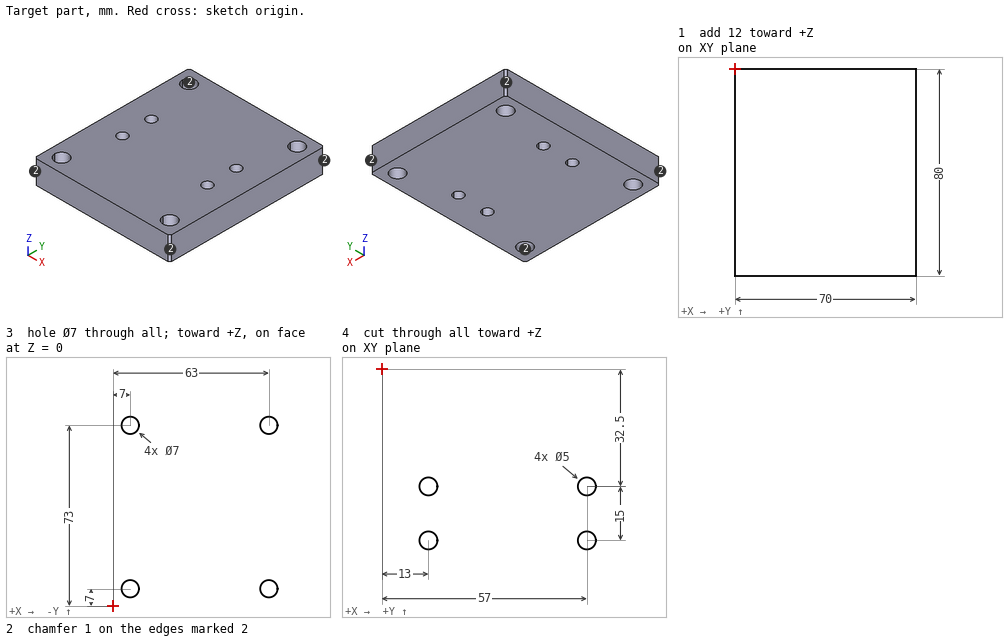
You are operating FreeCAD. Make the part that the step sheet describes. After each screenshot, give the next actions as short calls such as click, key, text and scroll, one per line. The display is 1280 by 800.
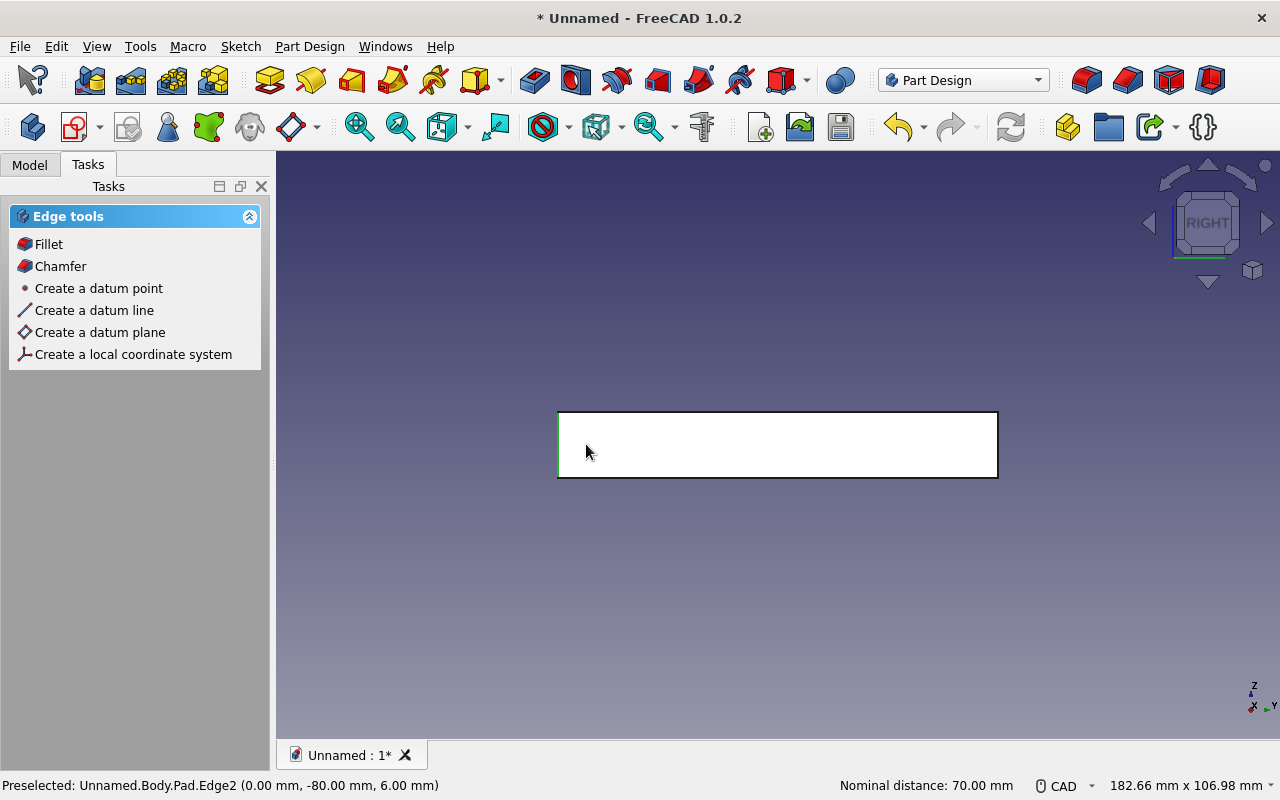
click(360, 128)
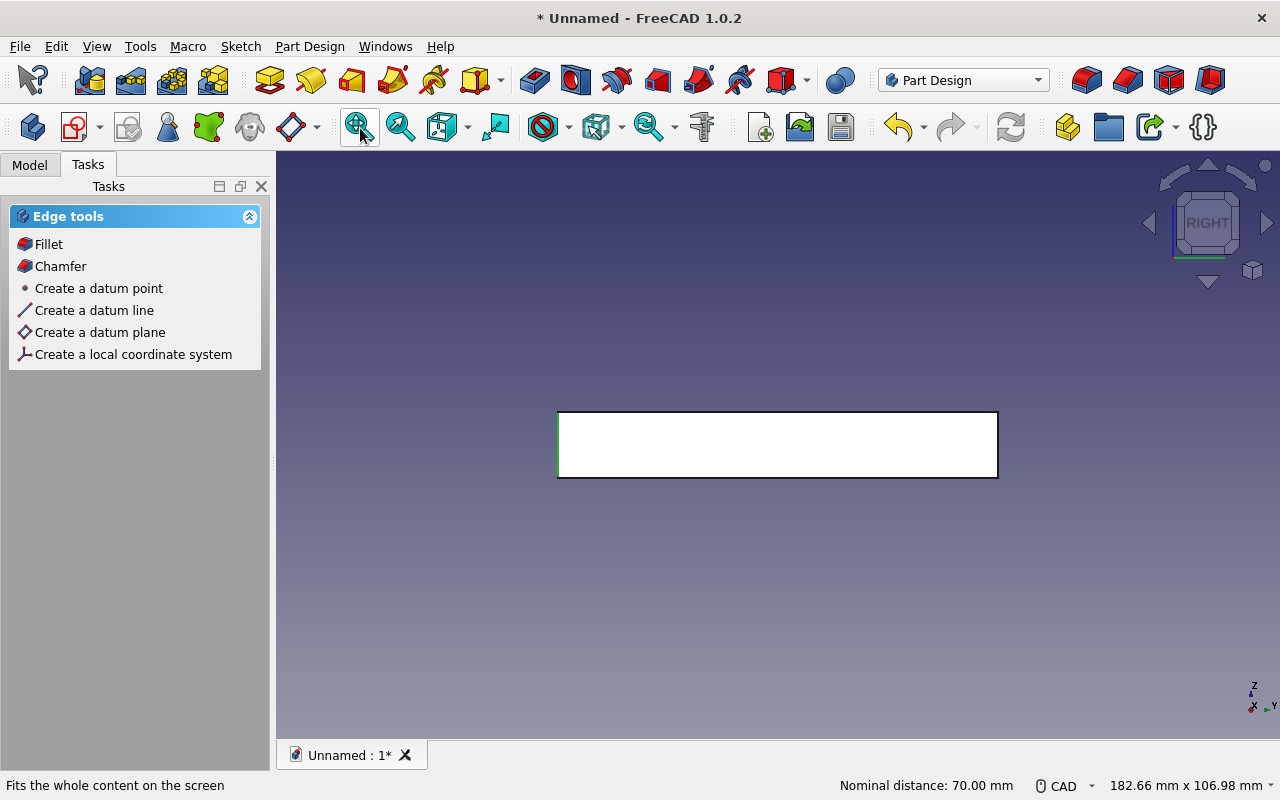
click(998, 444, ctrl)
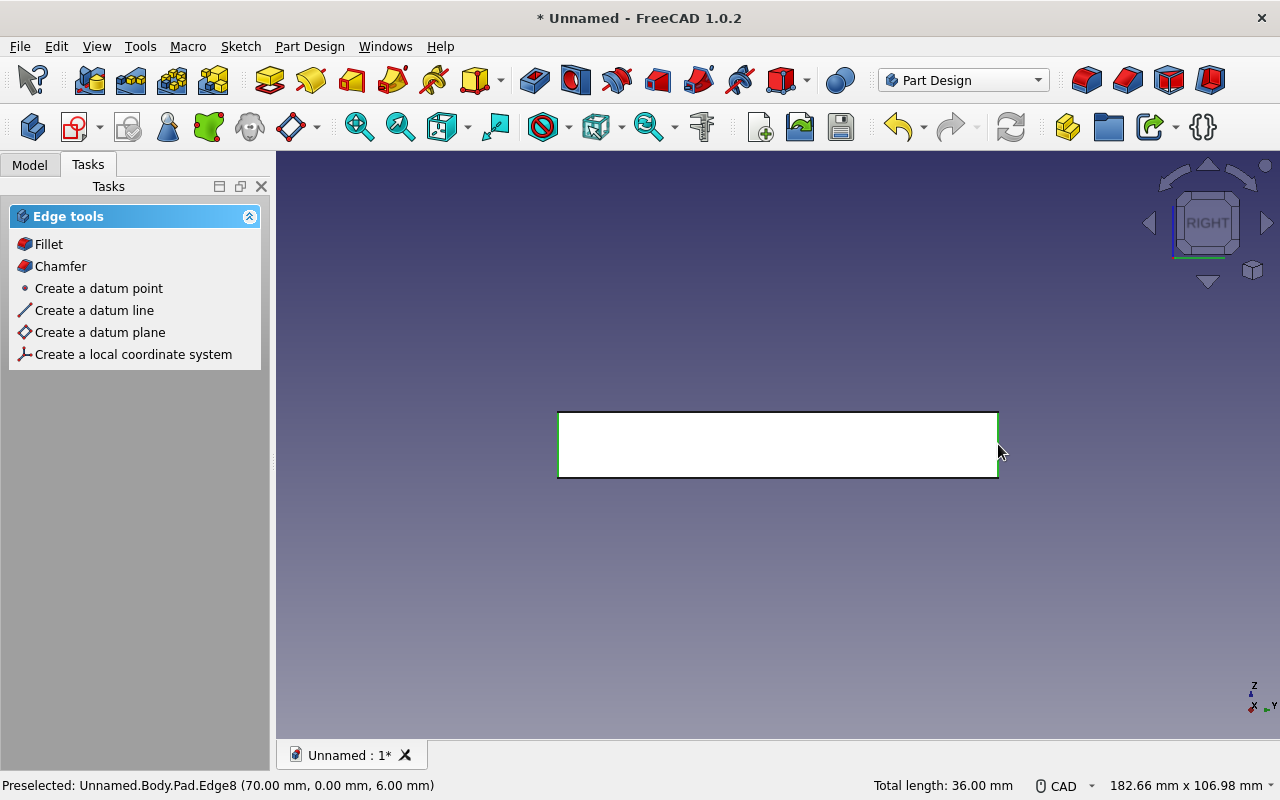
key(5)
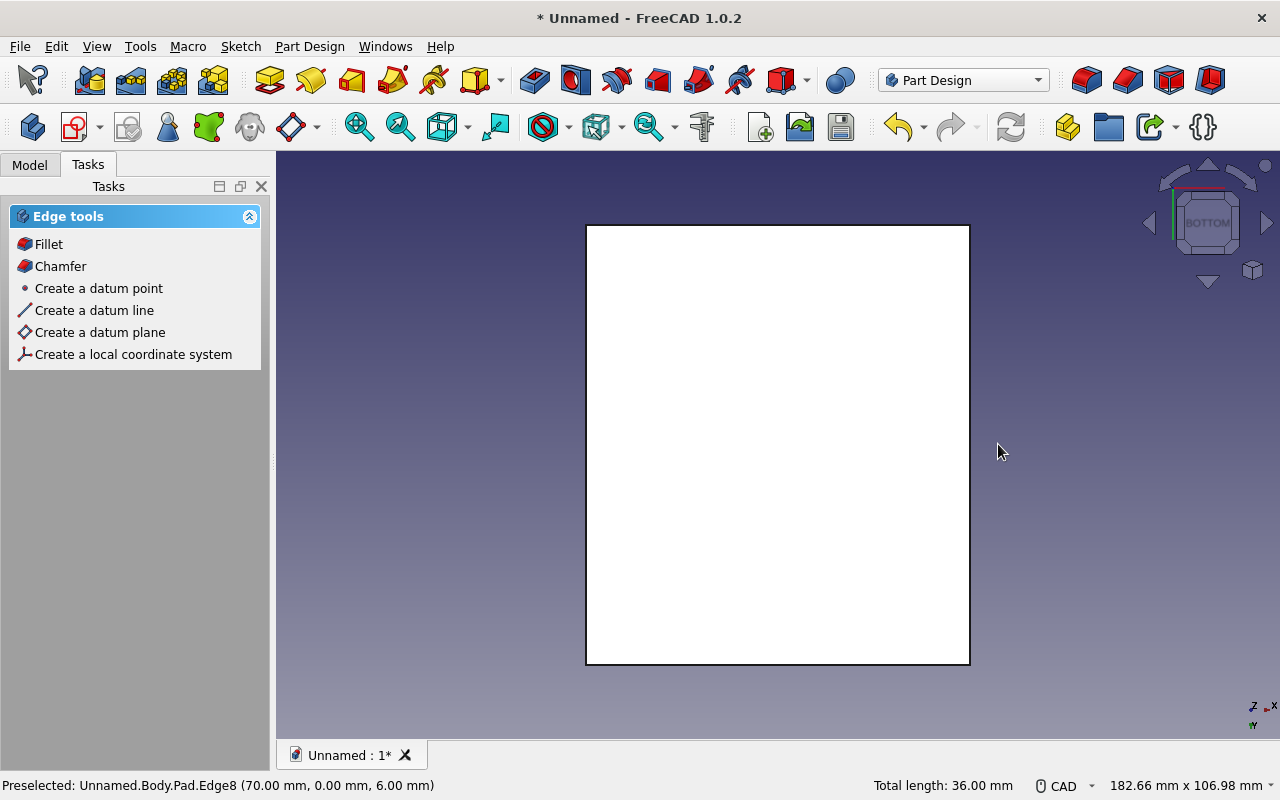
key(4)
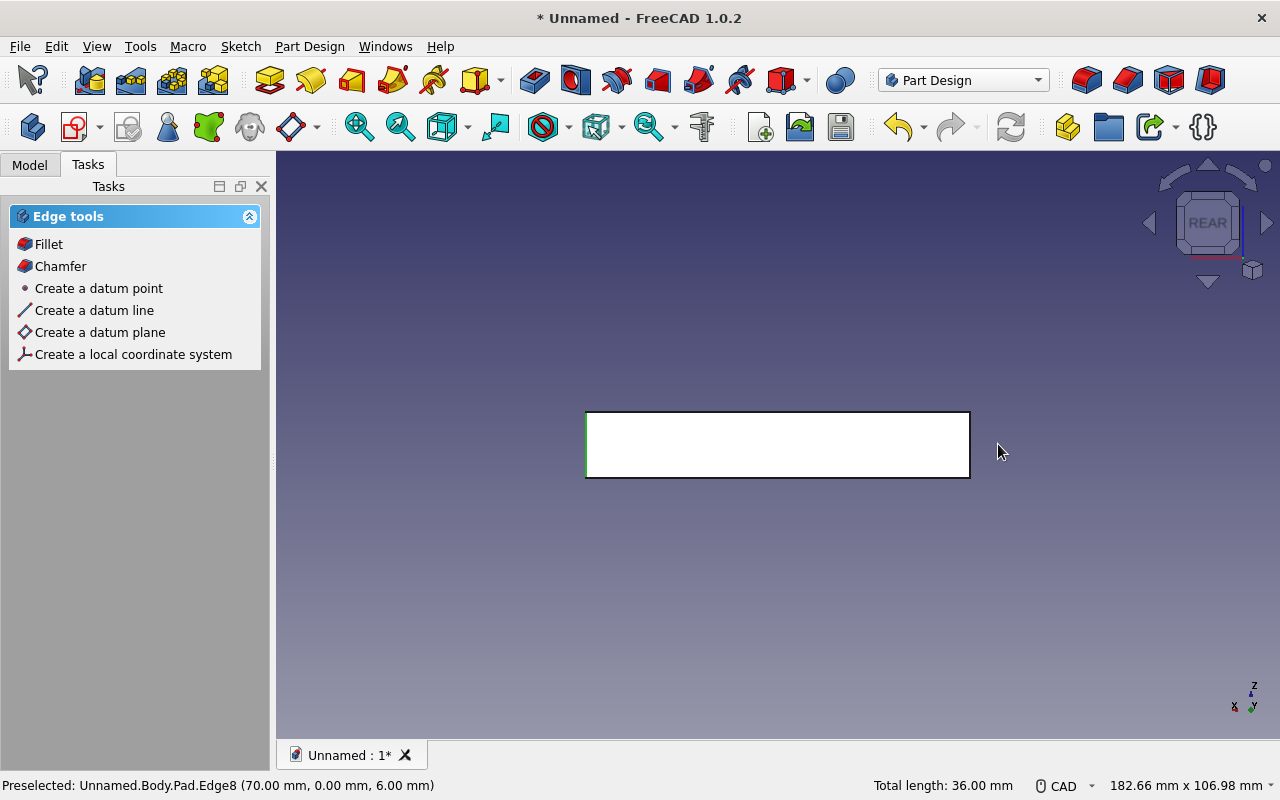
click(360, 128)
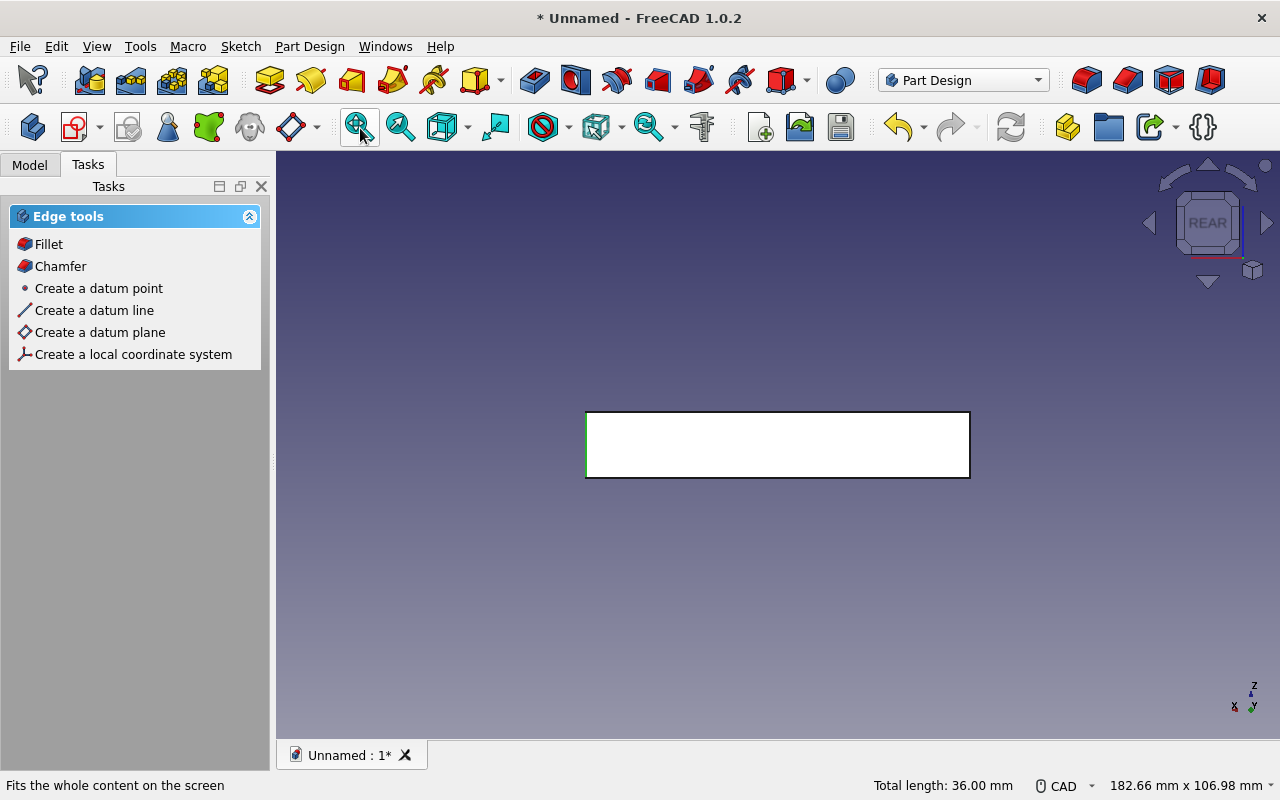
click(970, 444, ctrl)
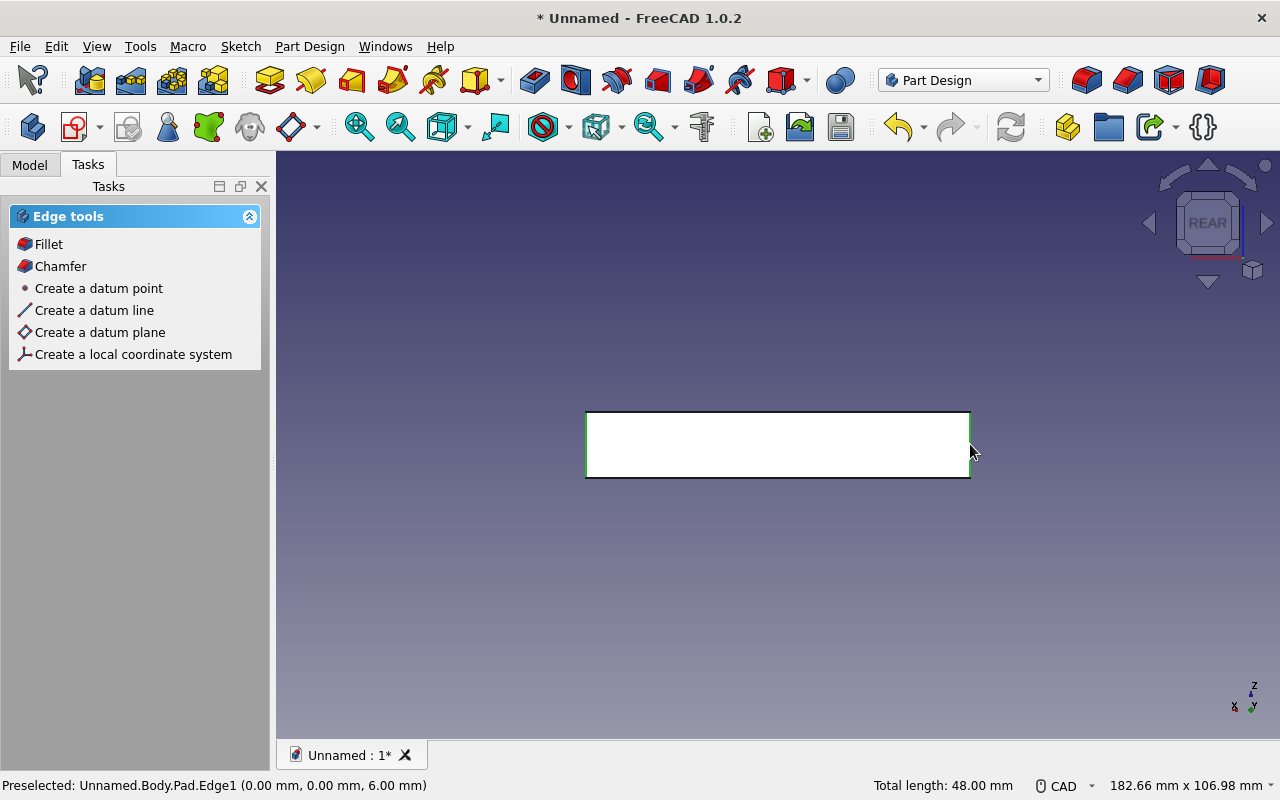
click(1128, 80)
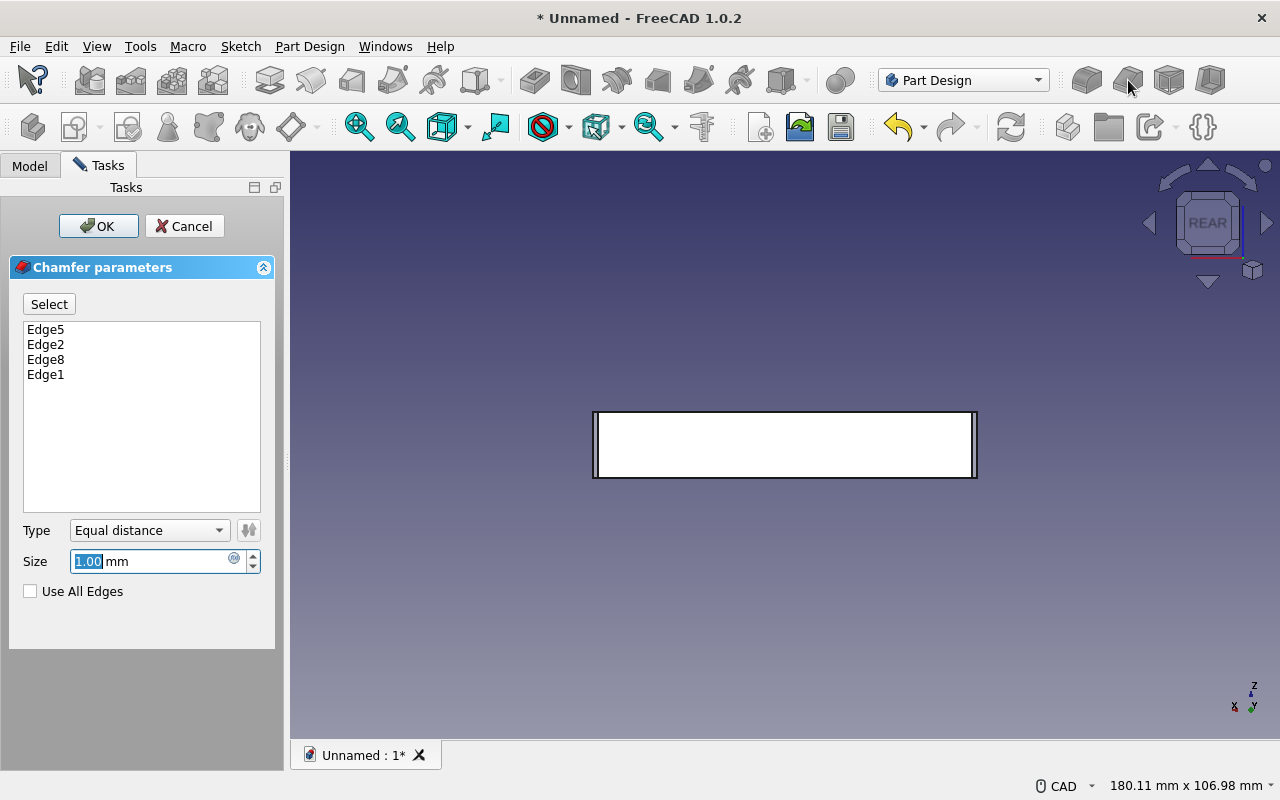
text(1)
key(Tab)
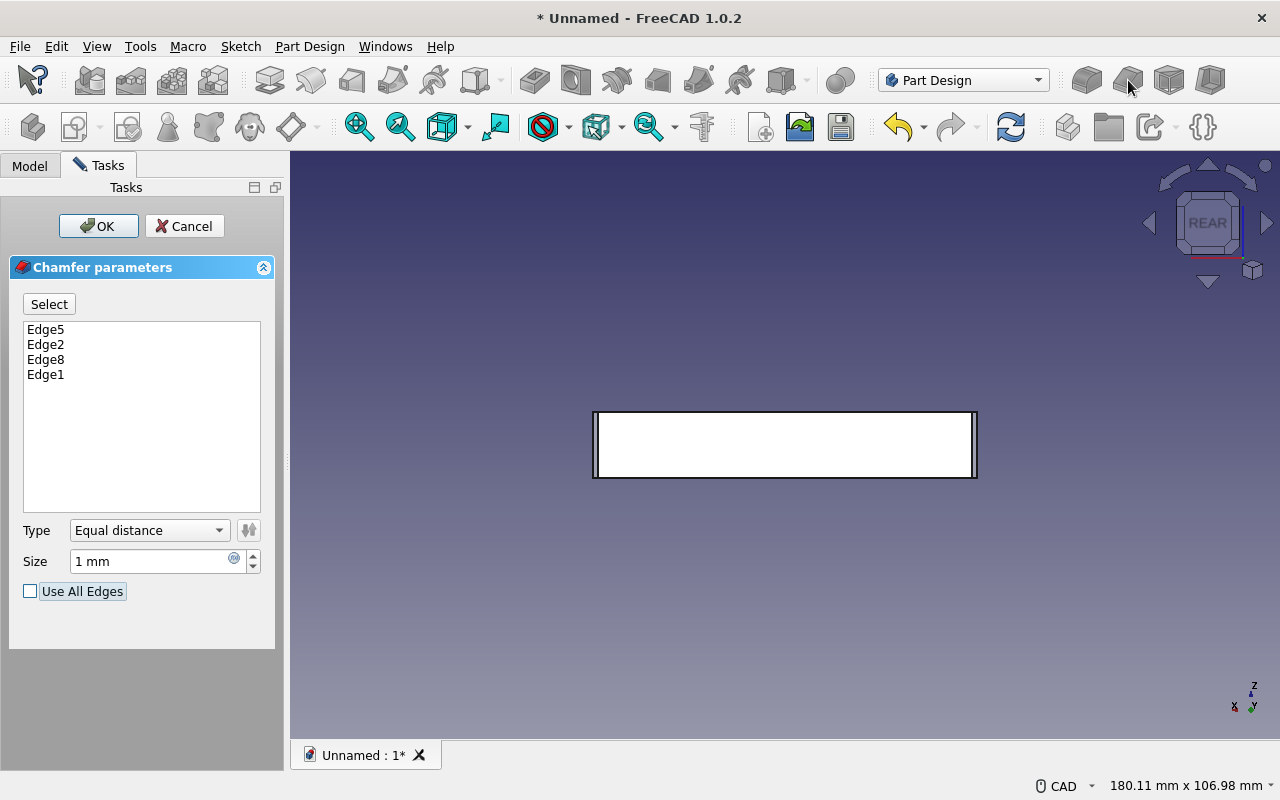
click(99, 226)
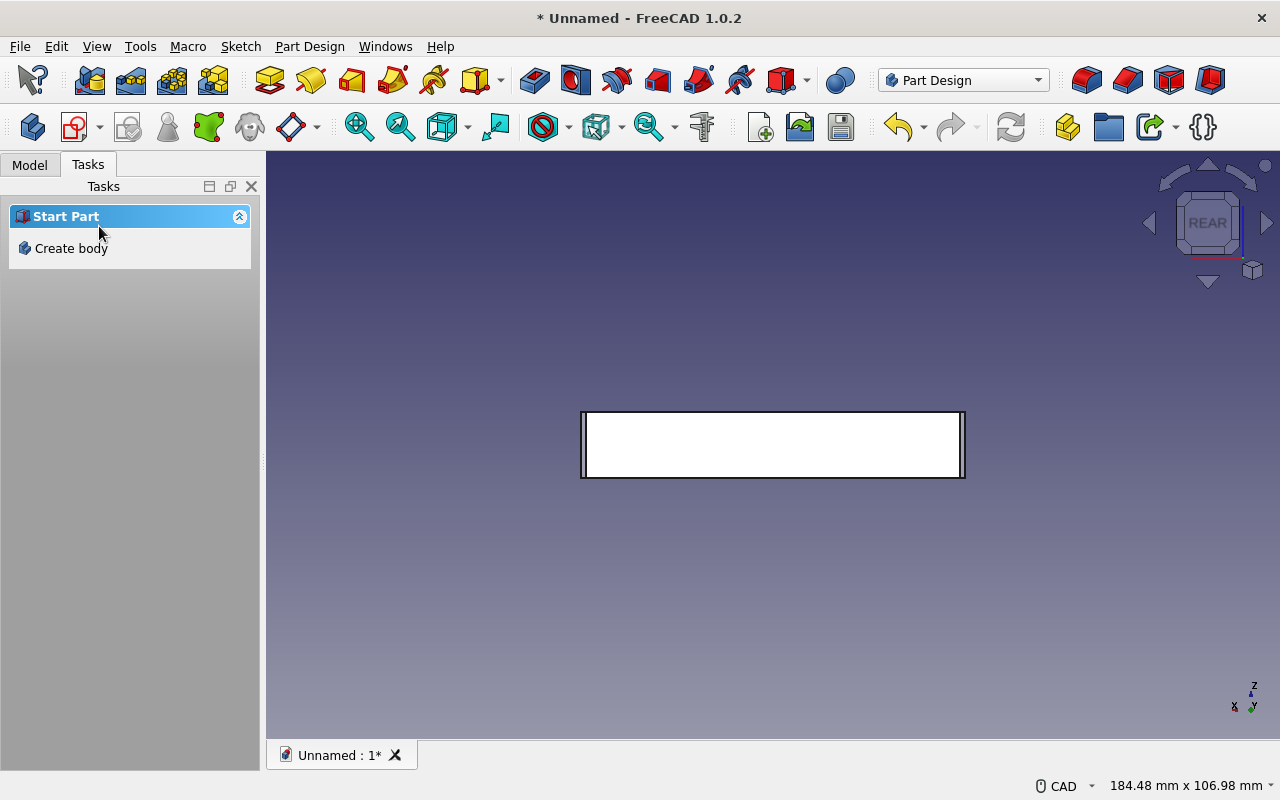
click(360, 128)